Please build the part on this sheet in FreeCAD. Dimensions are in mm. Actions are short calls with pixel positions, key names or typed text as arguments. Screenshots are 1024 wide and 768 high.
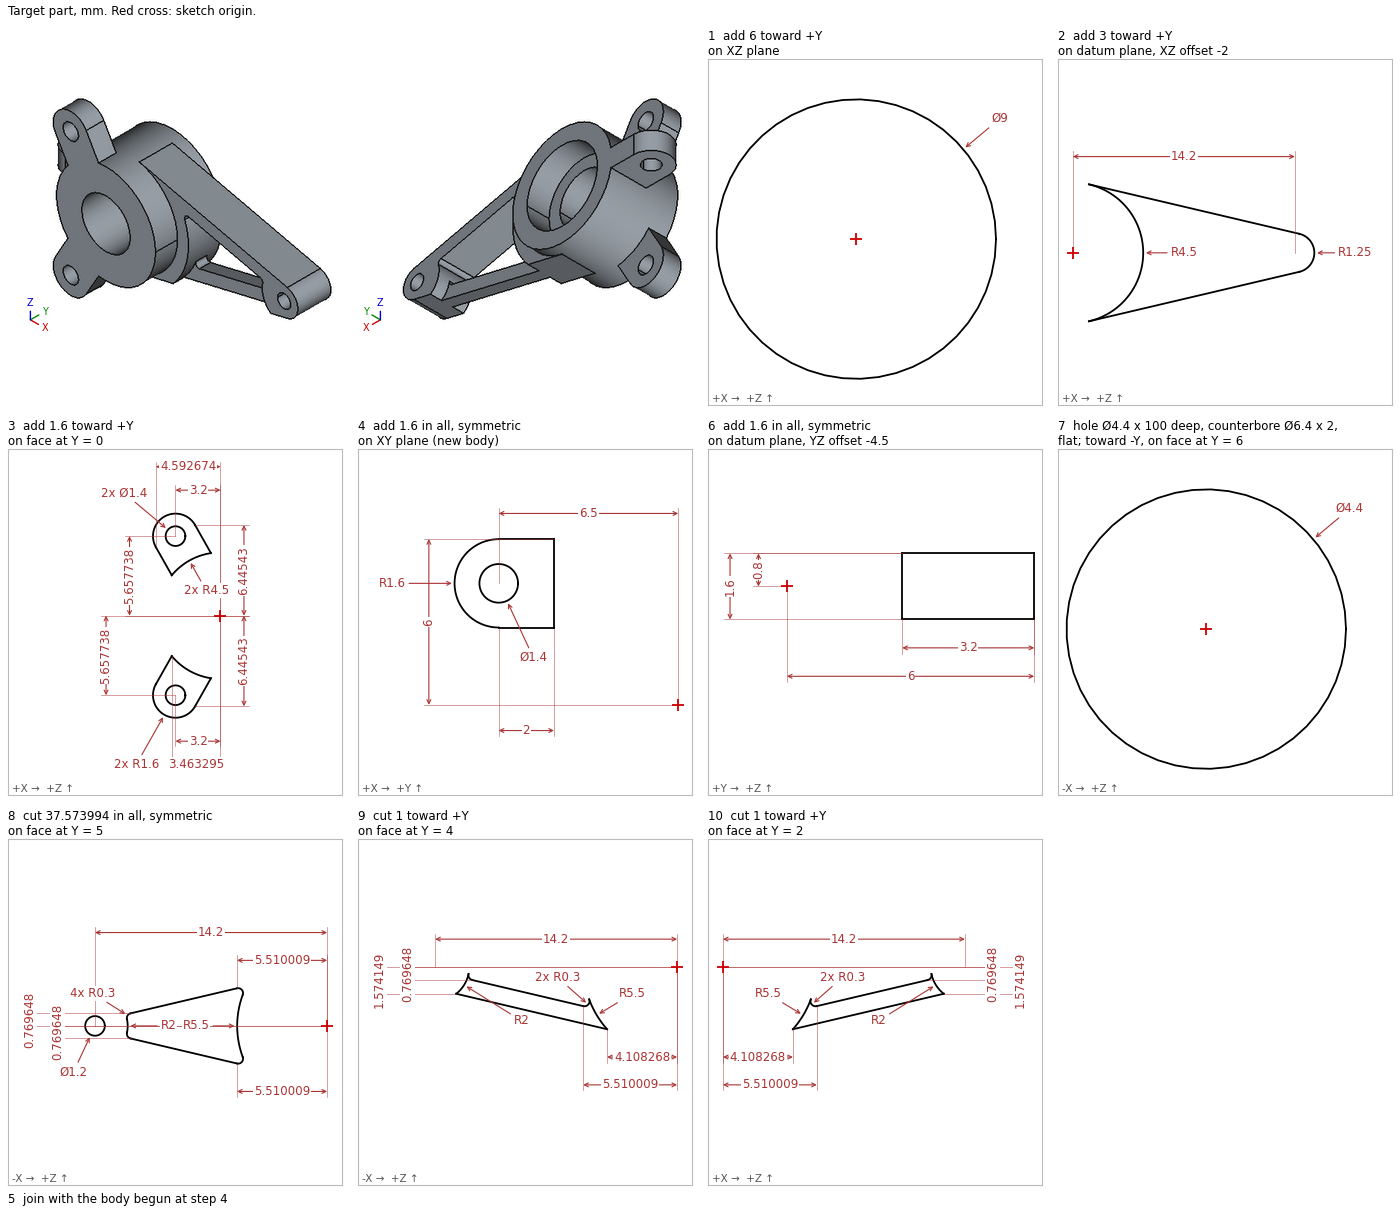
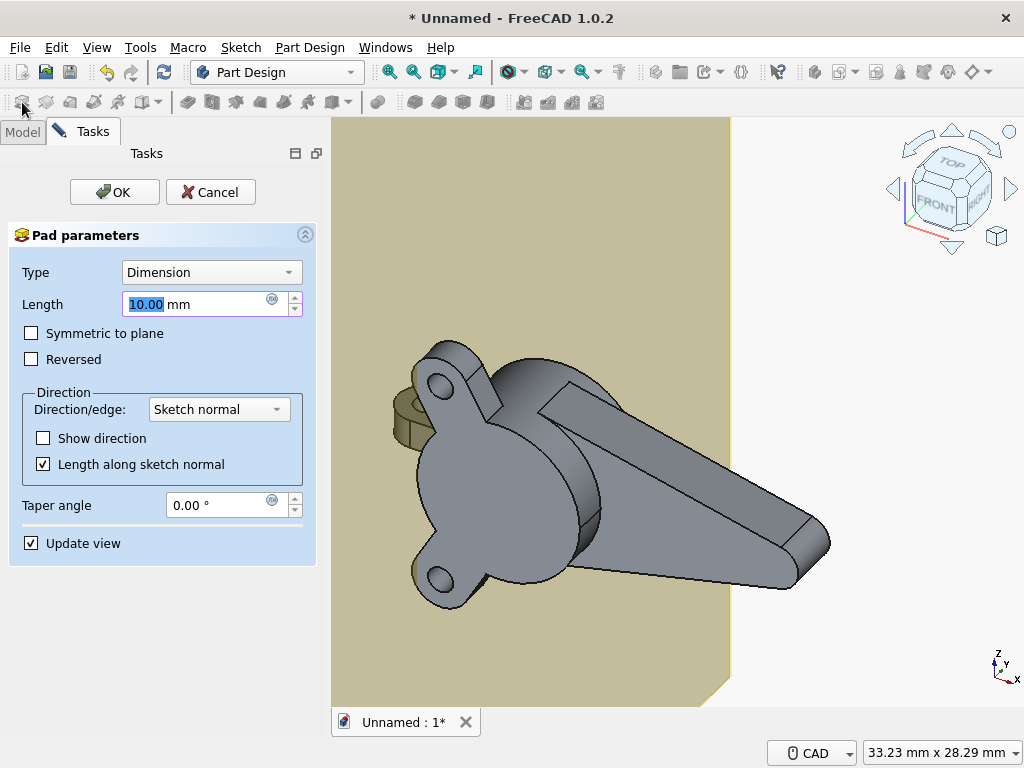
text(1.6)
key(Tab)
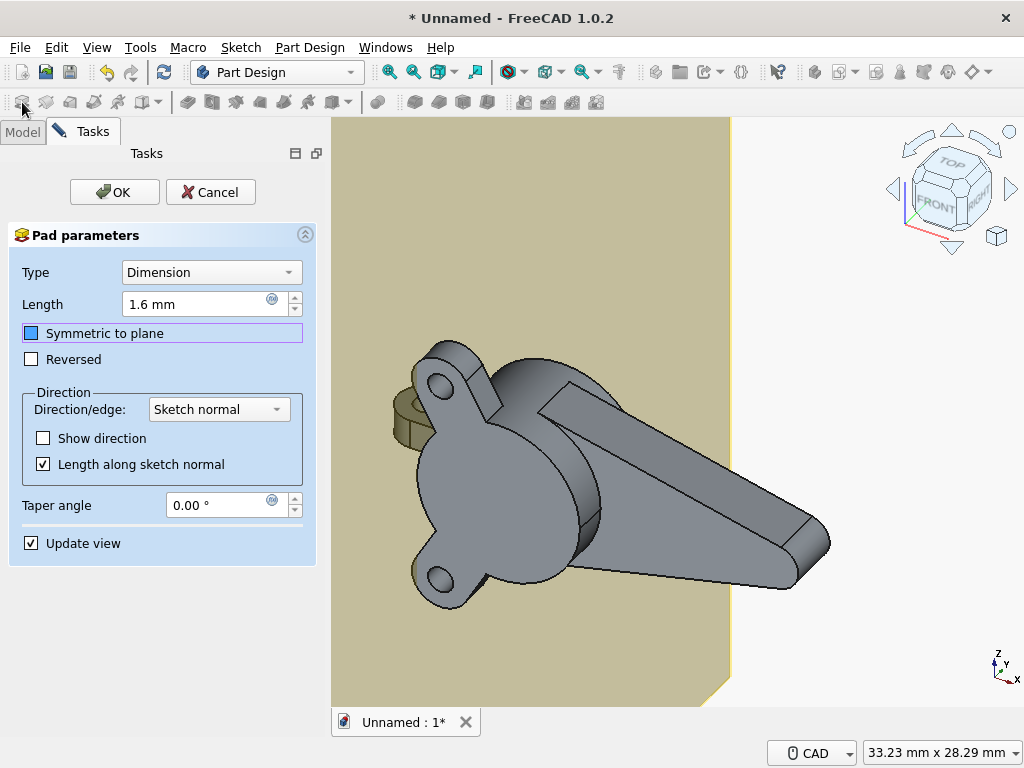
click(30, 333)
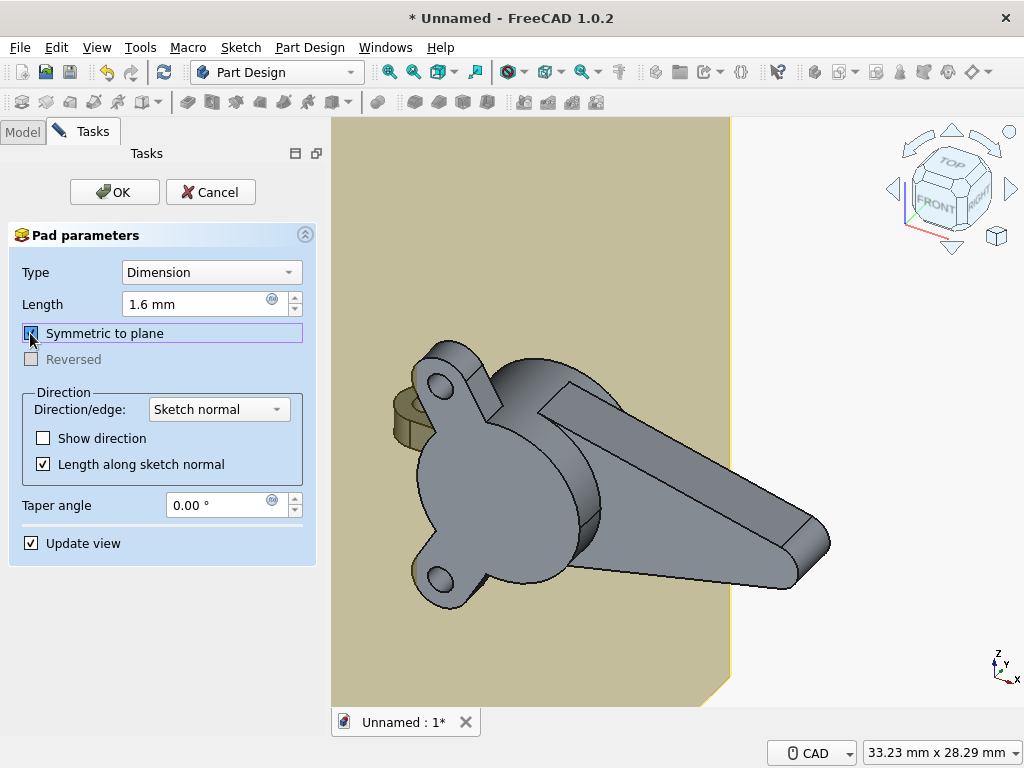
click(115, 192)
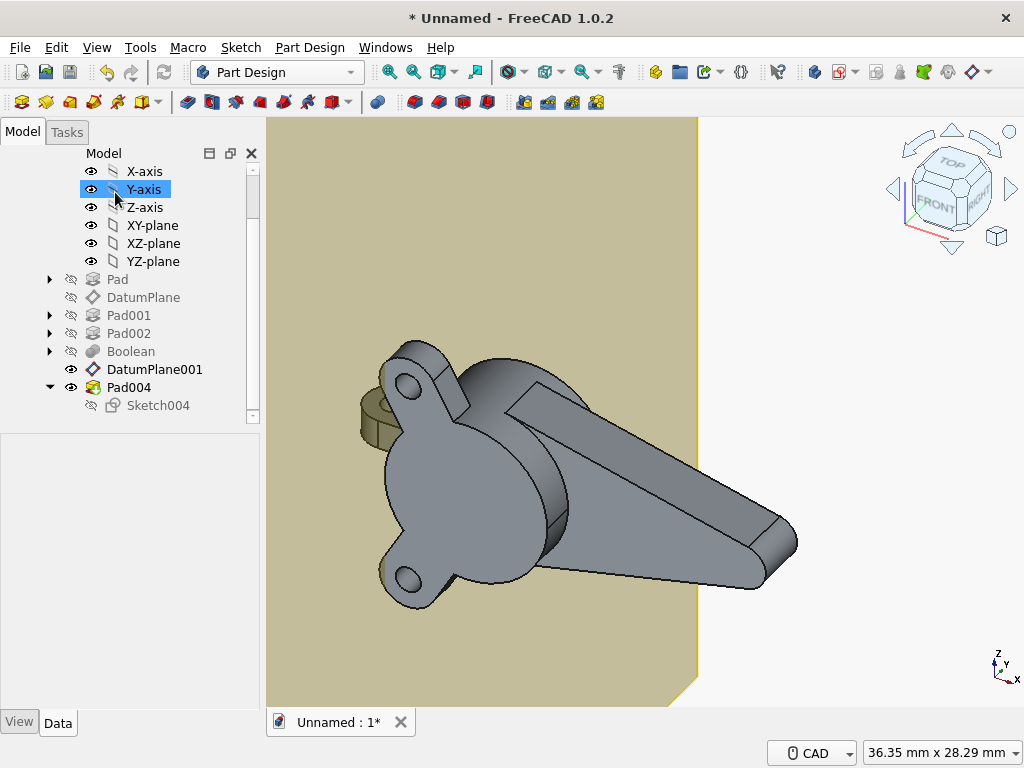
click(116, 369)
key(space)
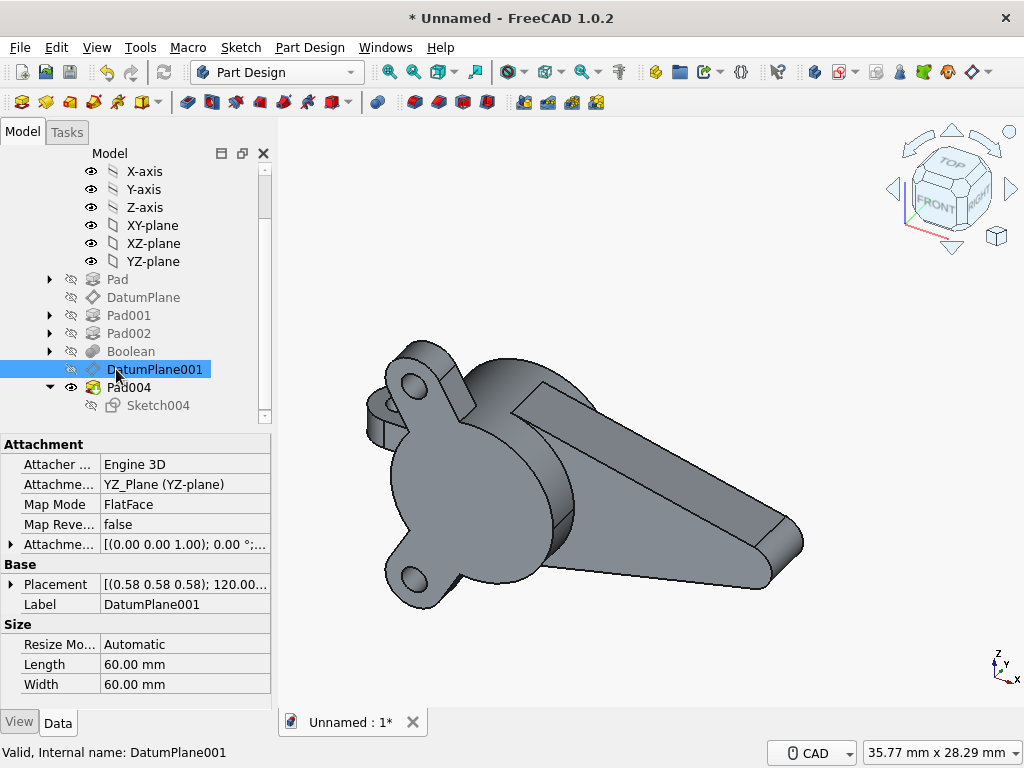
click(390, 72)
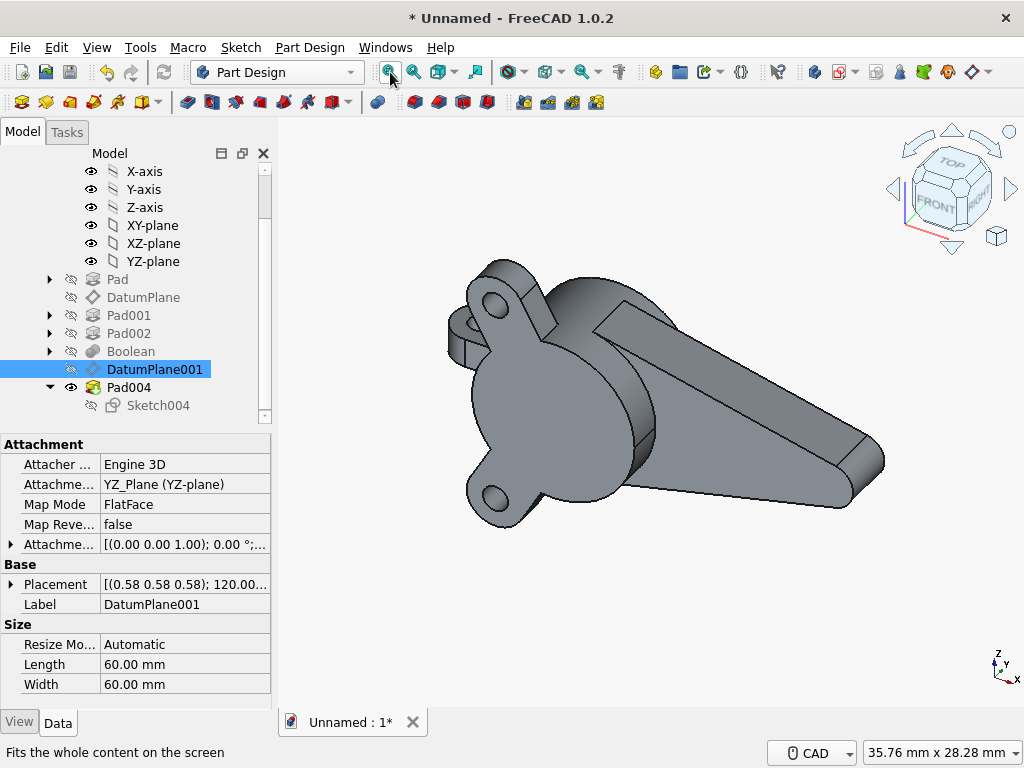
key(4)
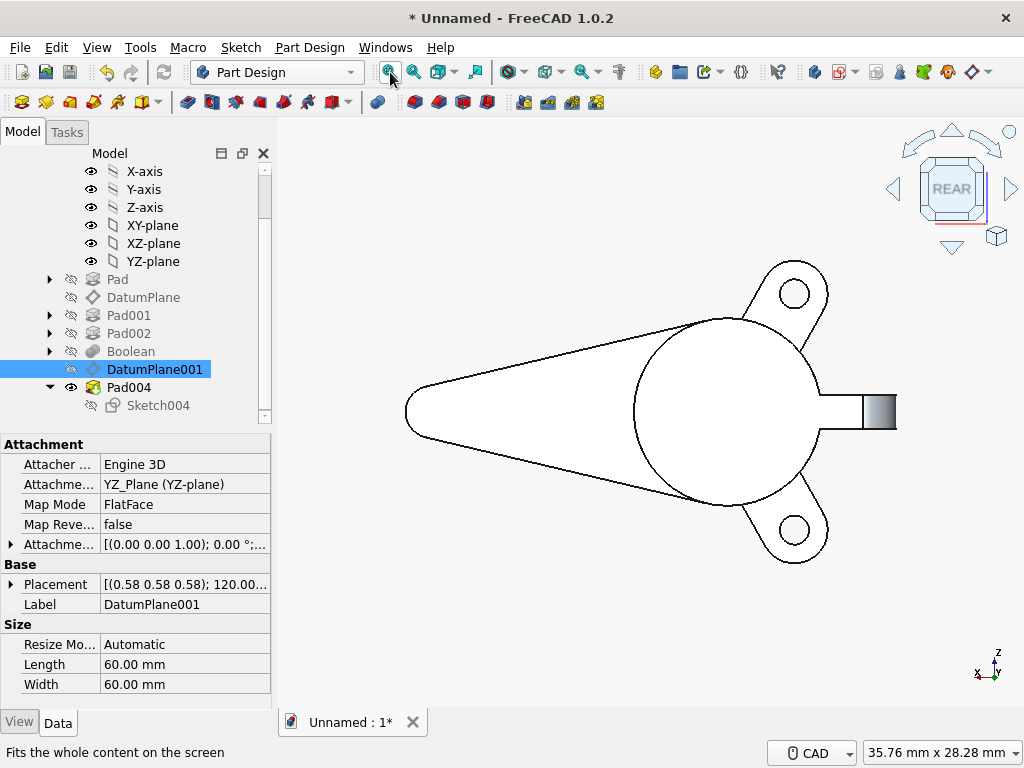
click(716, 411)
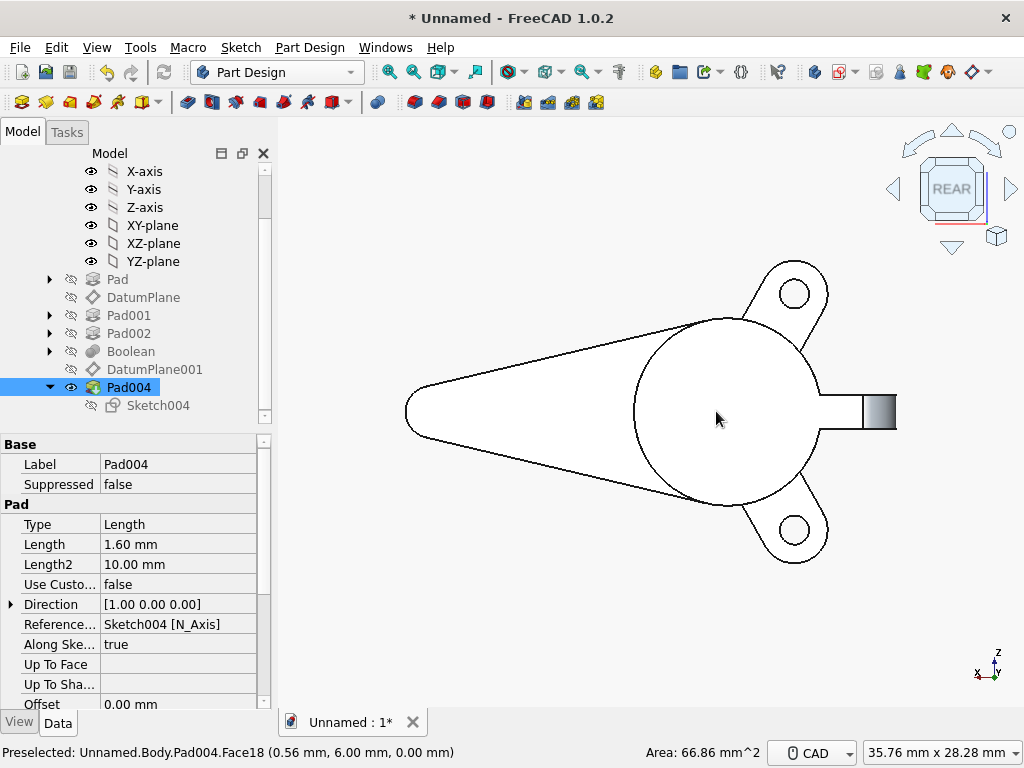
click(840, 72)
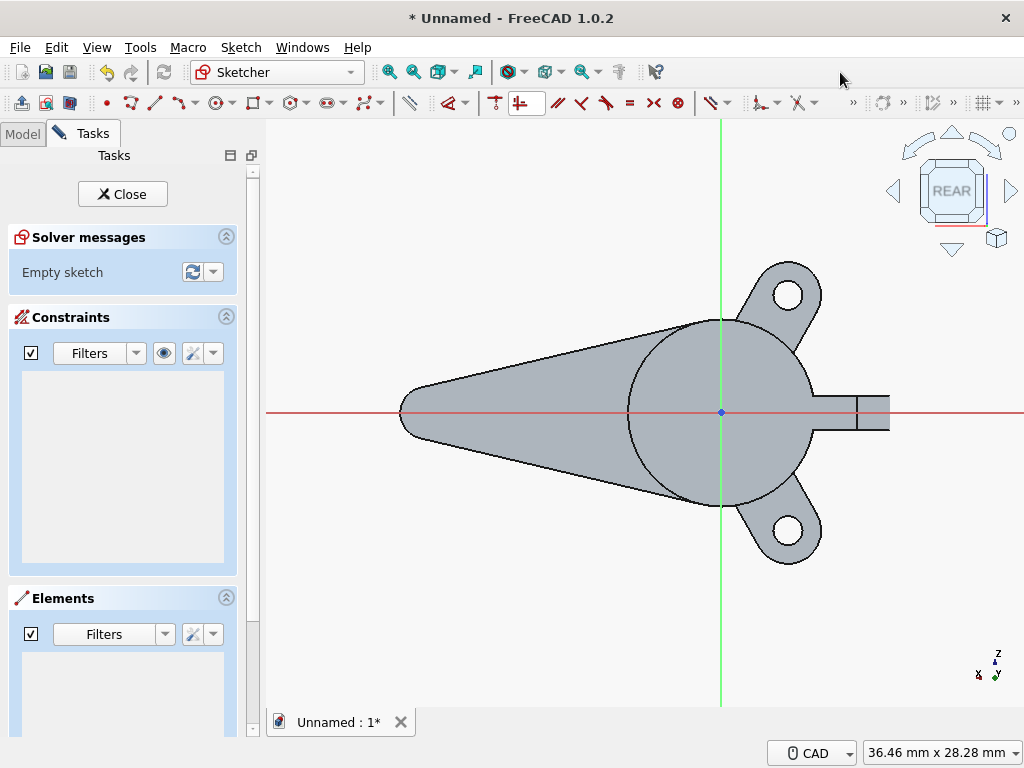
scroll(769, 413, up, 7)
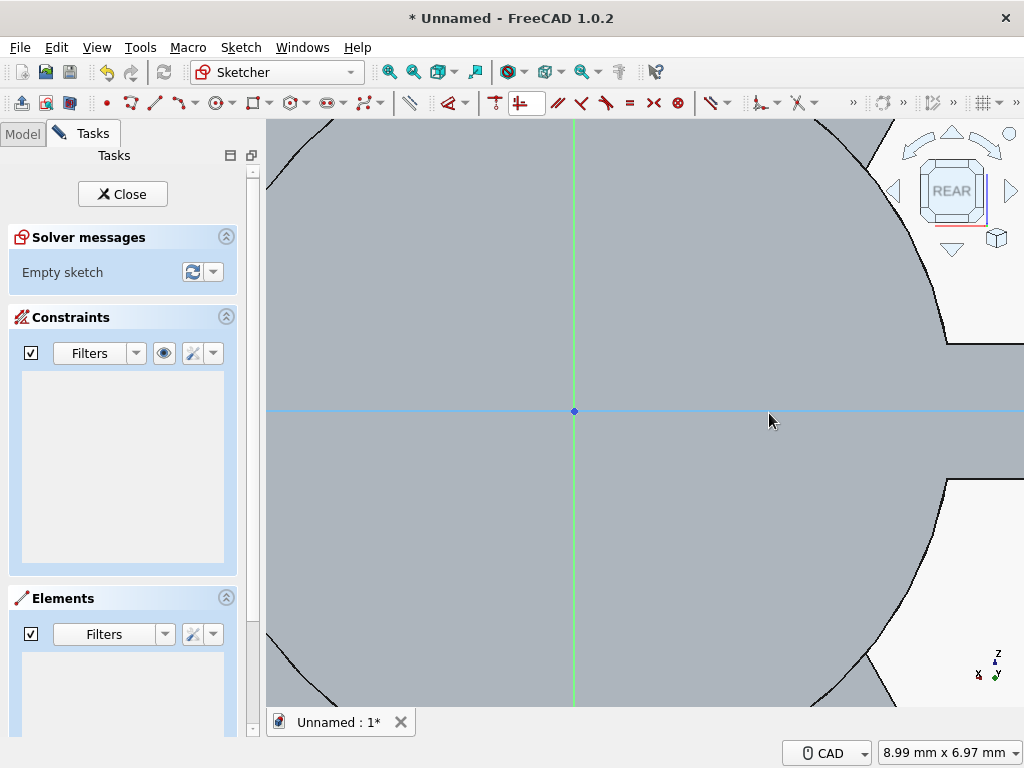
key(g)
key(c)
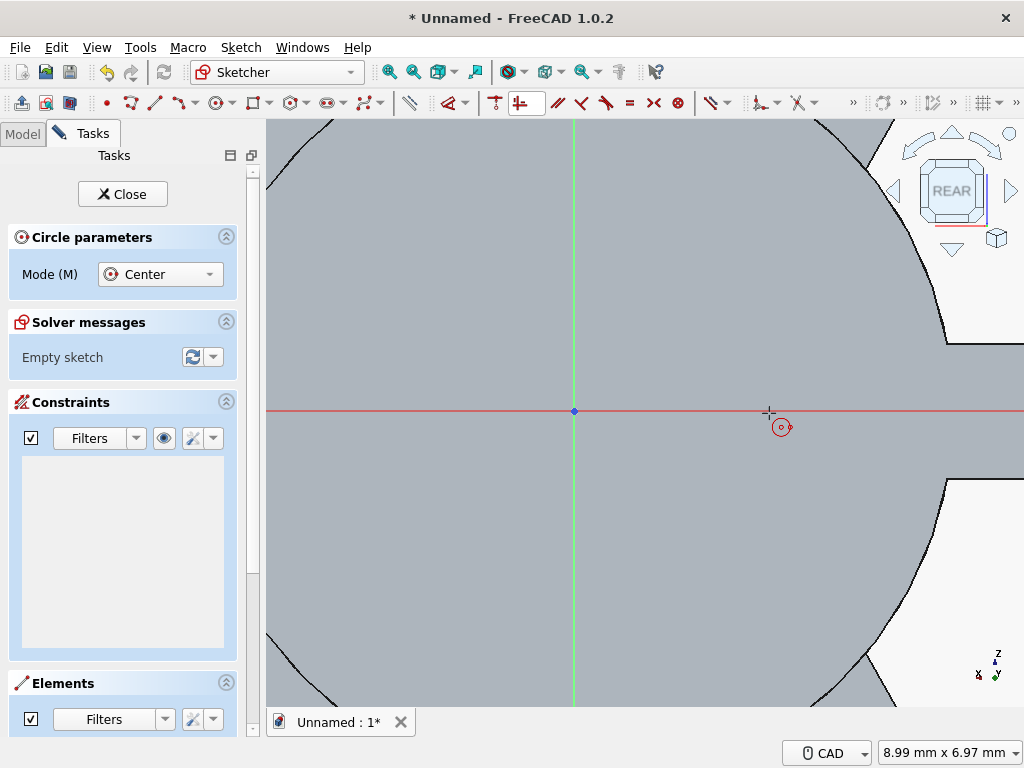
click(574, 411)
click(705, 280)
key(Escape)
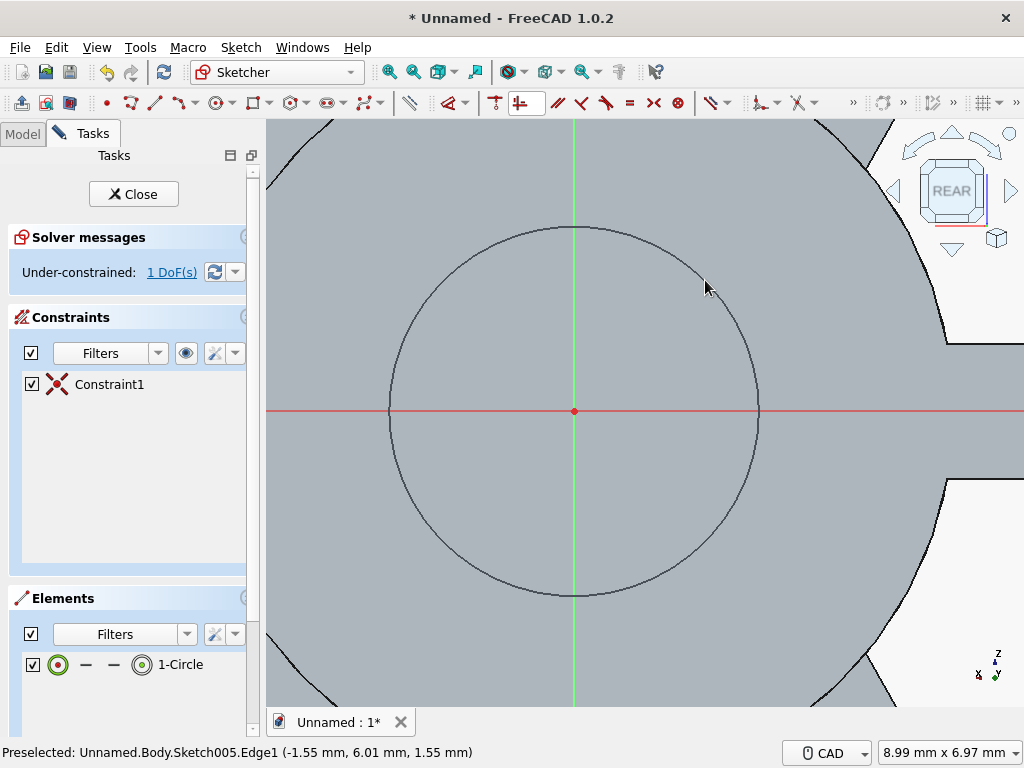
key(d)